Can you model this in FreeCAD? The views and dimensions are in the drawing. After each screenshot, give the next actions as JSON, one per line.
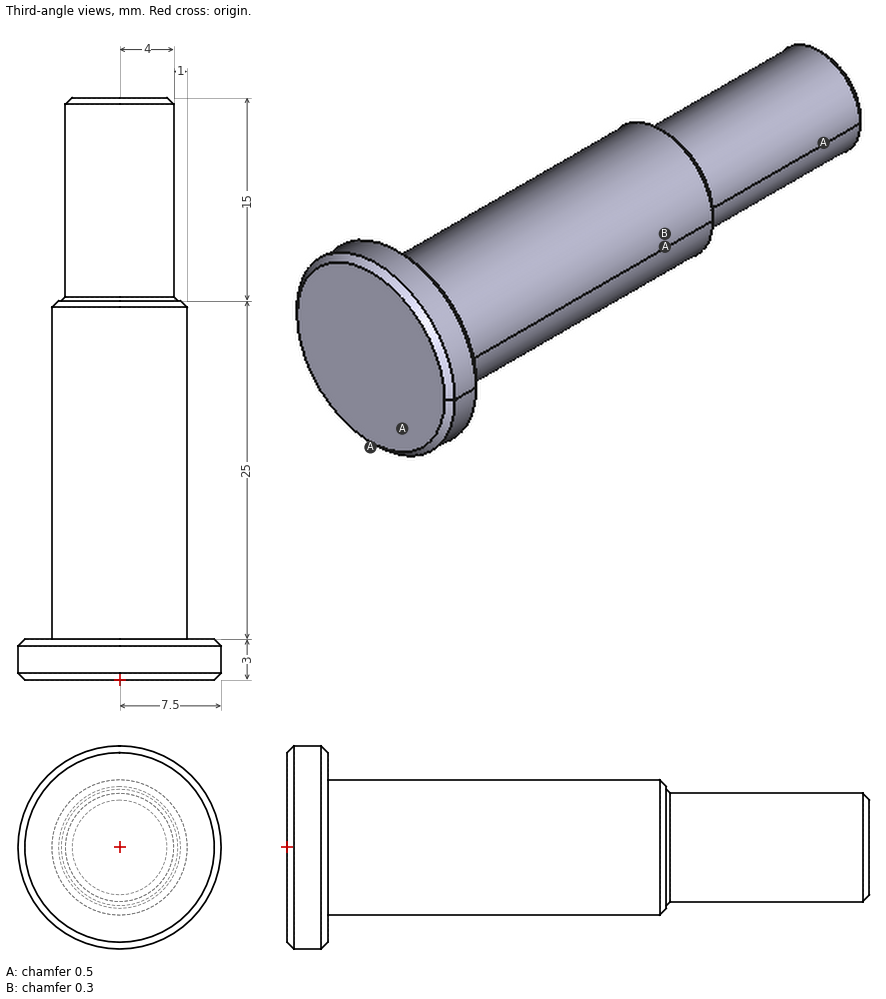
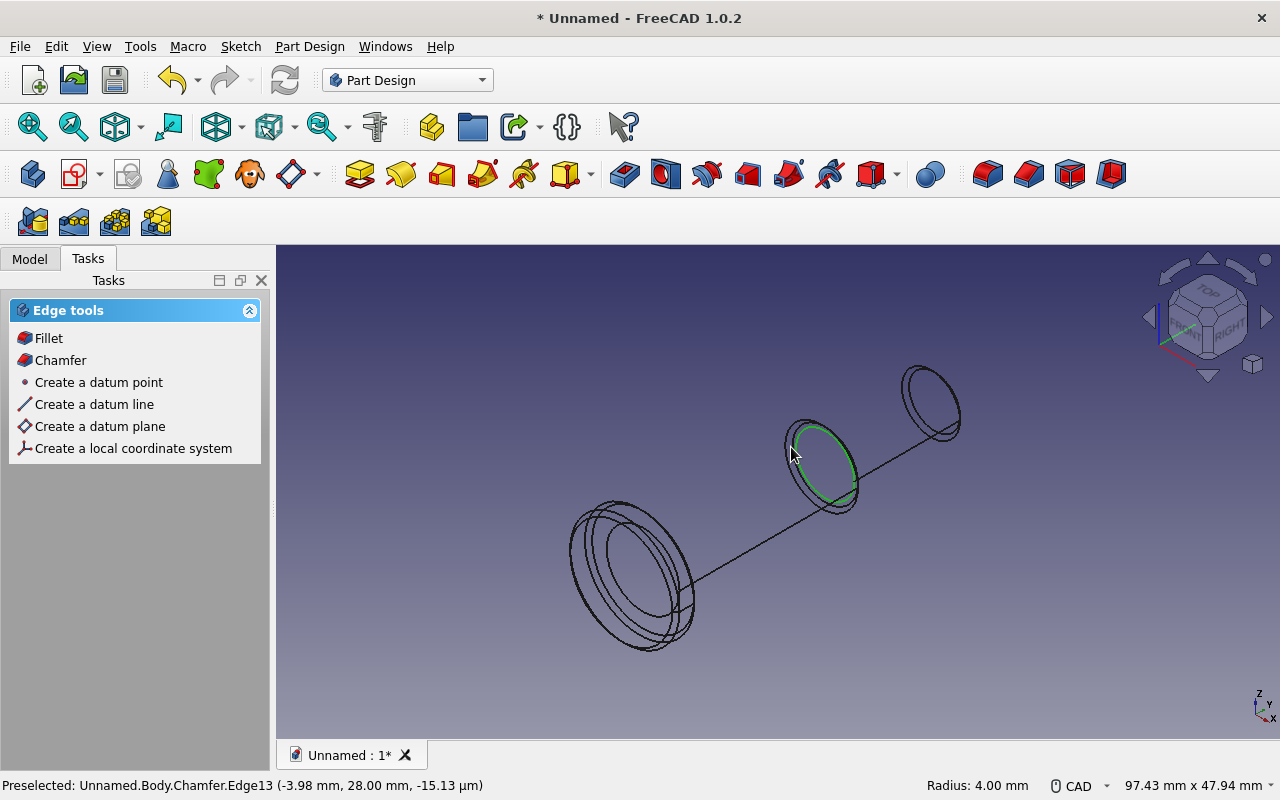
{"action": "key", "text": "v 1"}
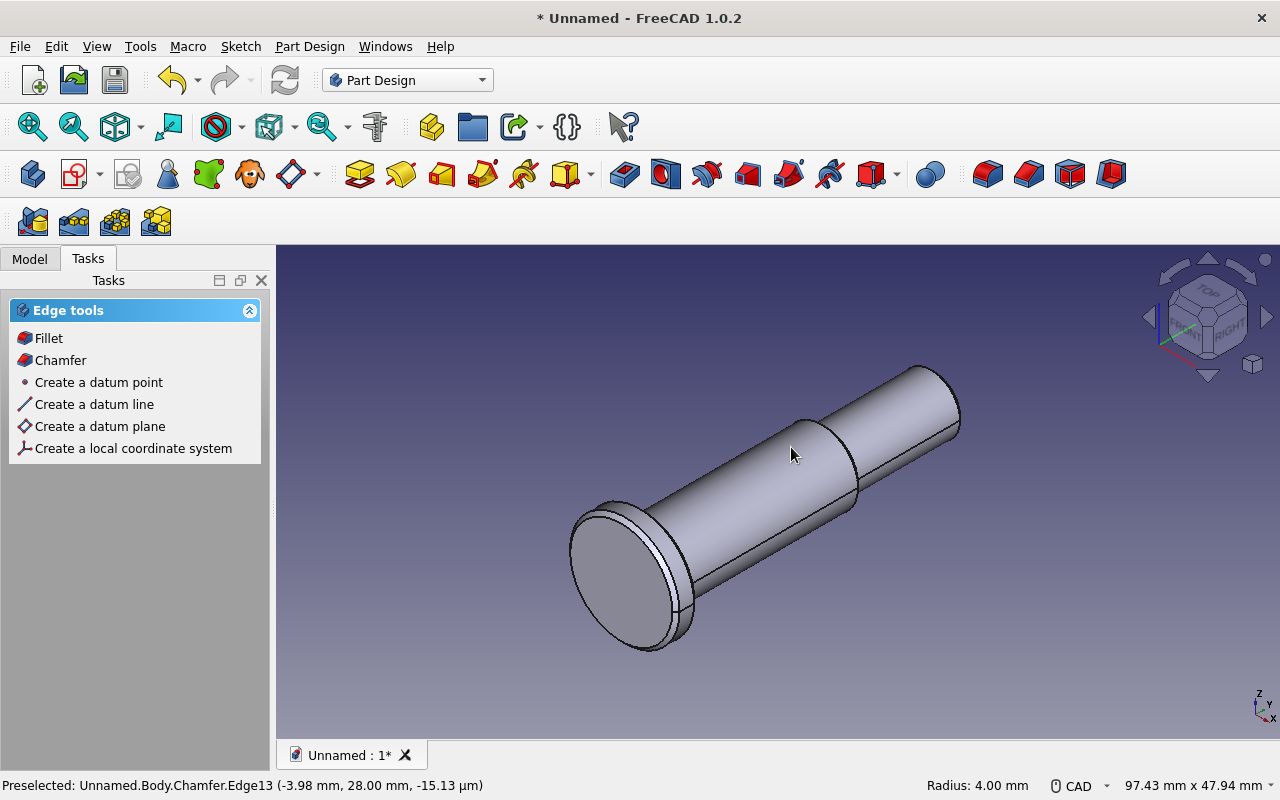
{"action": "left_click", "coordinate": [1029, 174]}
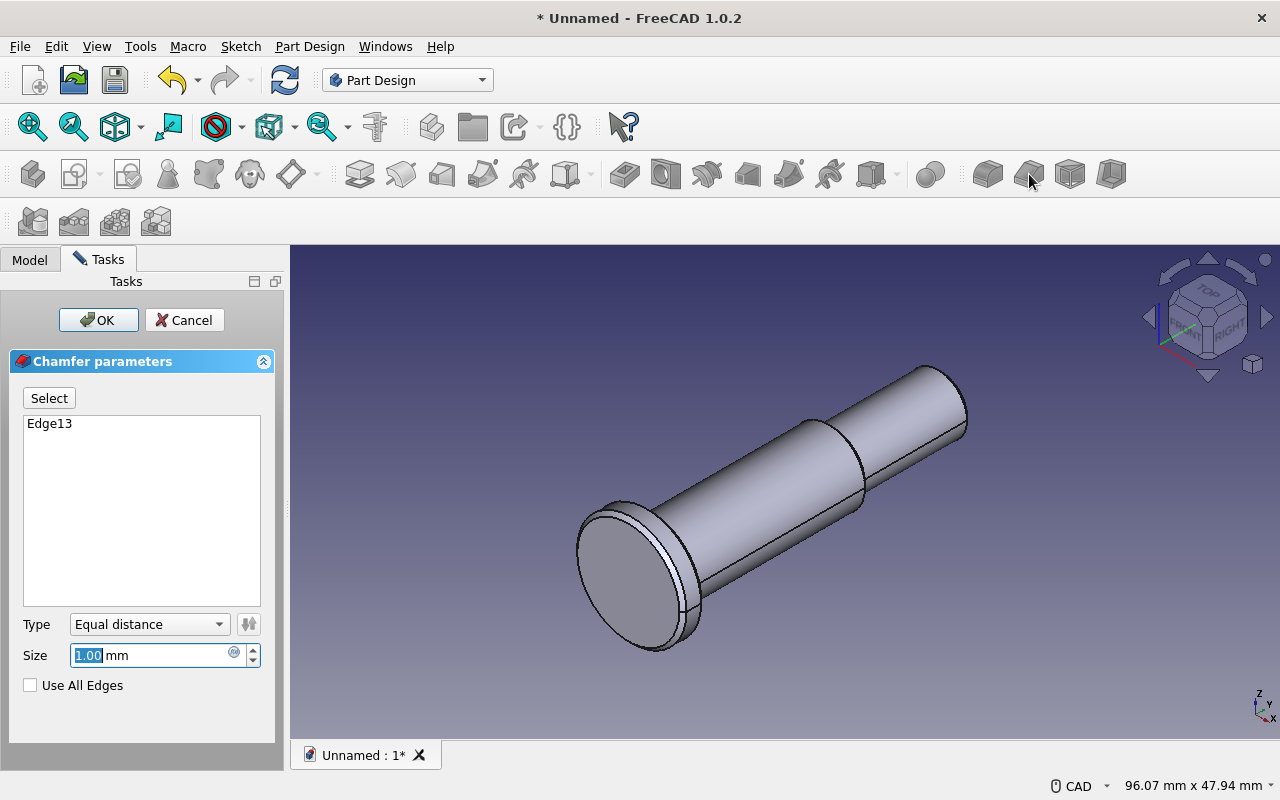
{"action": "type", "text": "0.3"}
{"action": "key", "text": "Tab"}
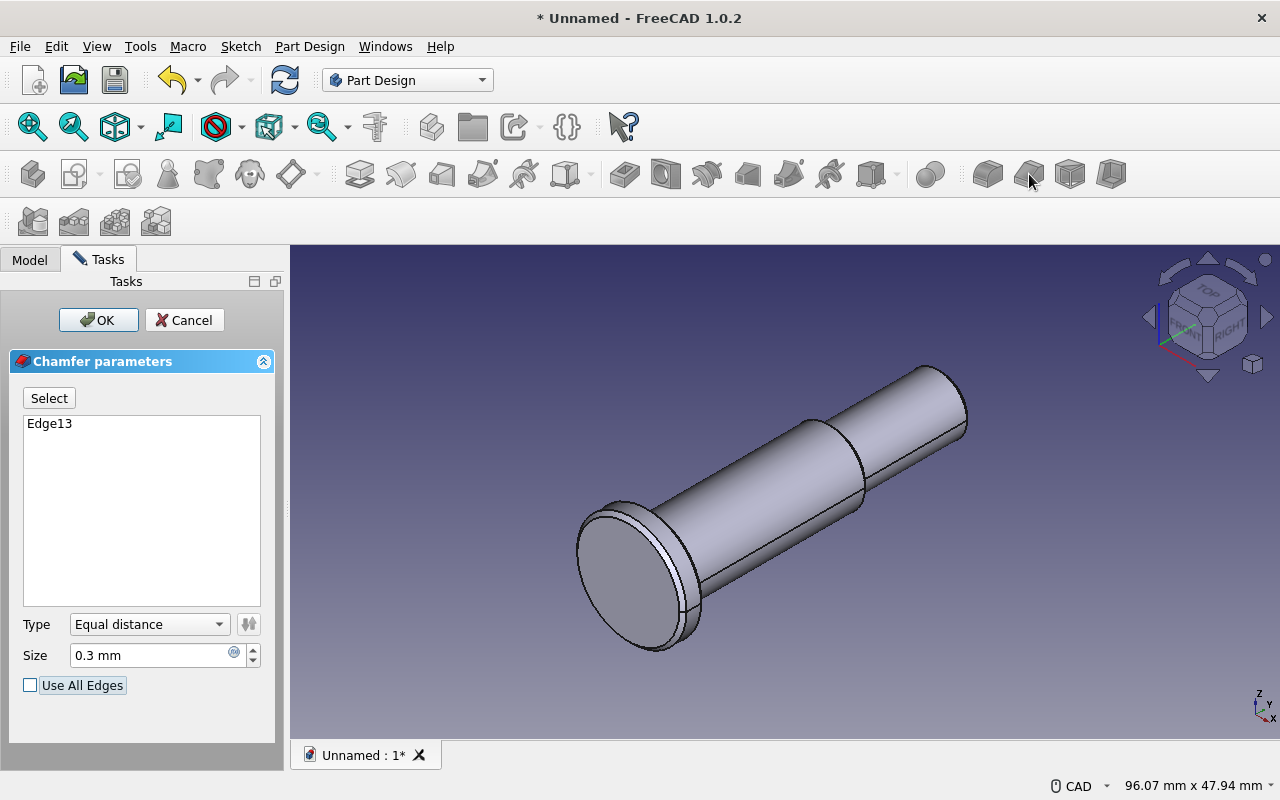
{"action": "left_click", "coordinate": [99, 320]}